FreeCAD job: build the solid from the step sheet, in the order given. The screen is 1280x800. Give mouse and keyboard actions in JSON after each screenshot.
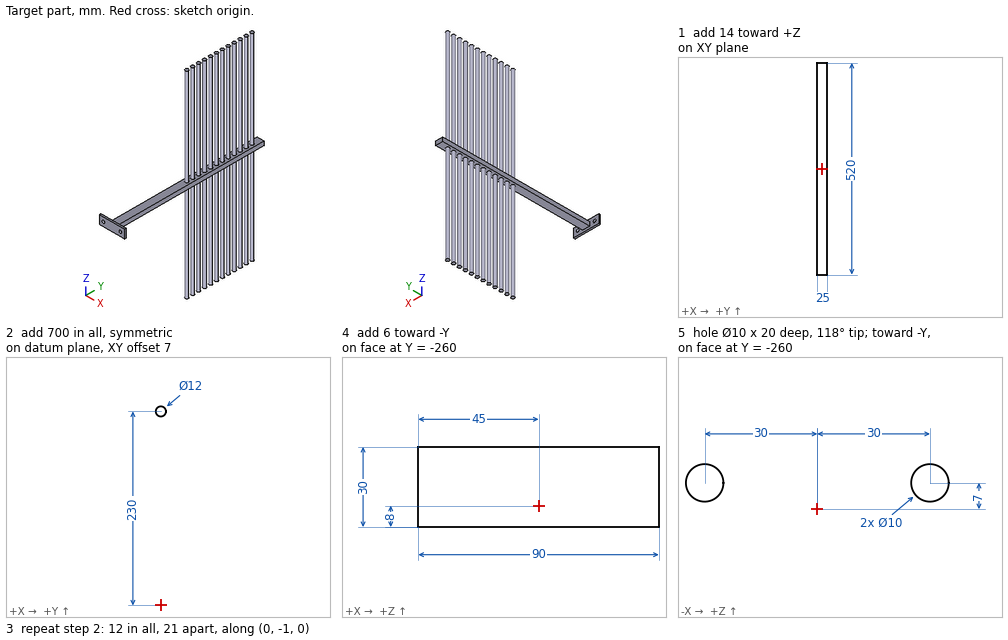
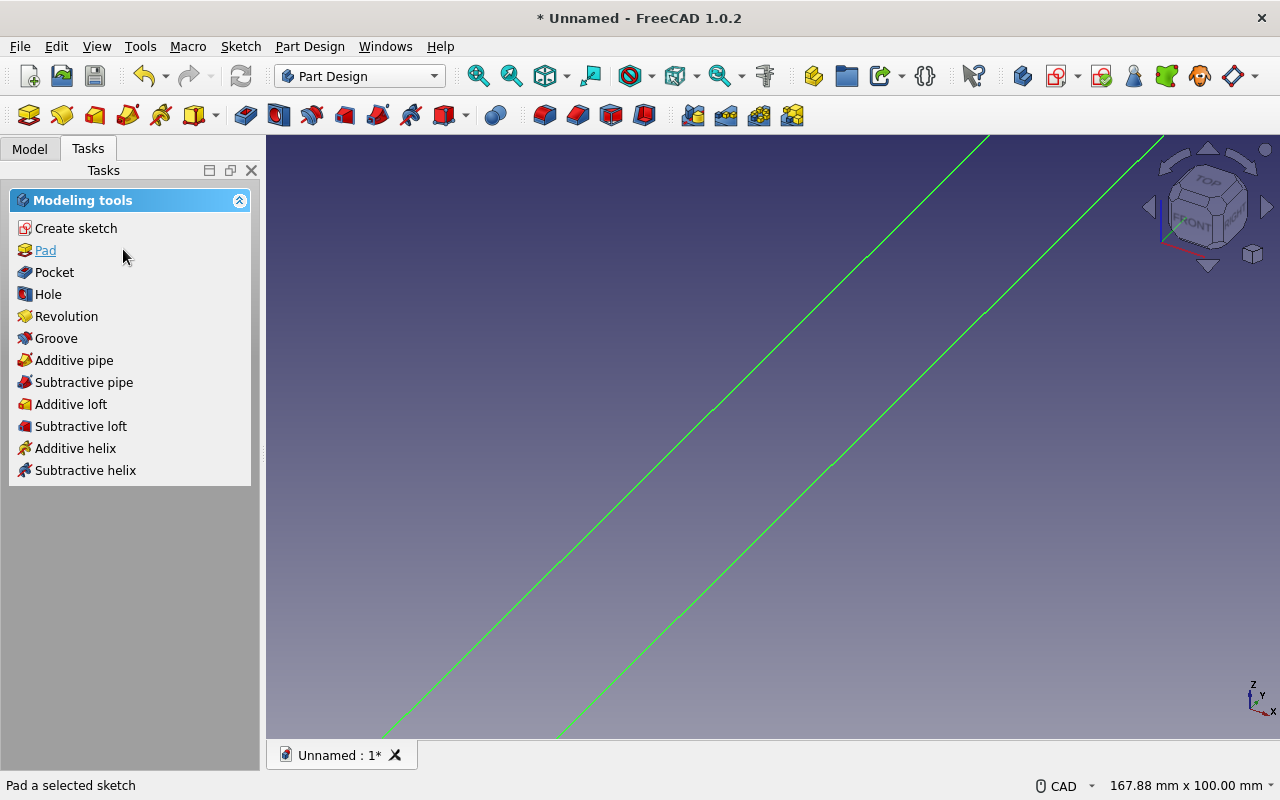
{"action": "left_click", "coordinate": [29, 116]}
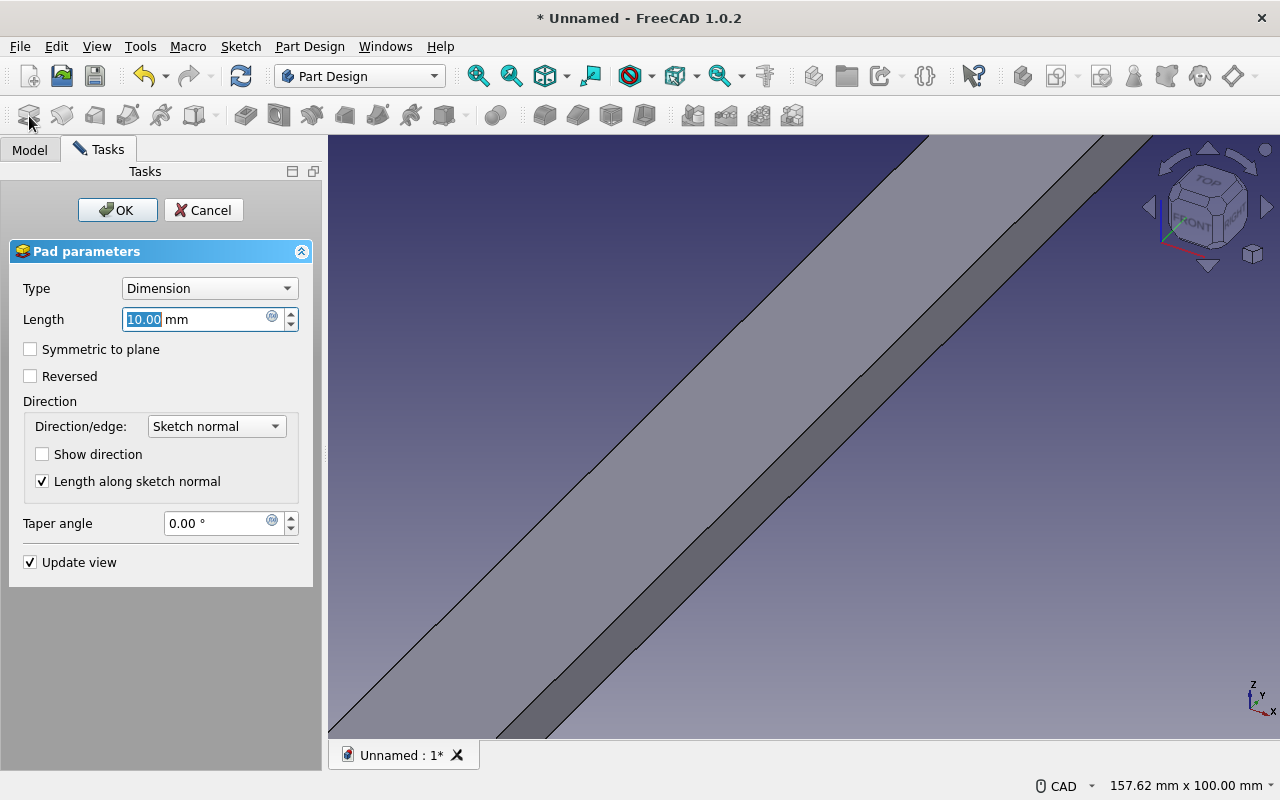
{"action": "type", "text": "14"}
{"action": "key", "text": "Tab"}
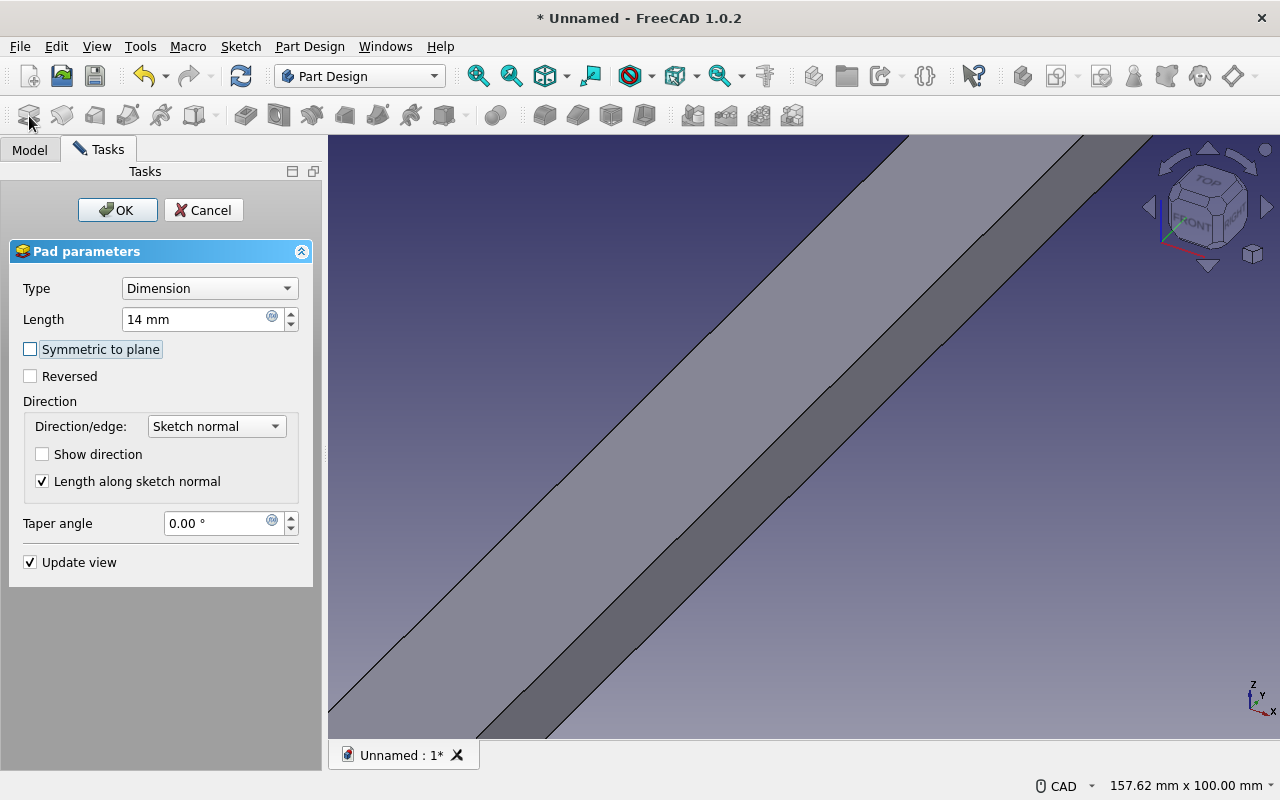
{"action": "left_click", "coordinate": [118, 210]}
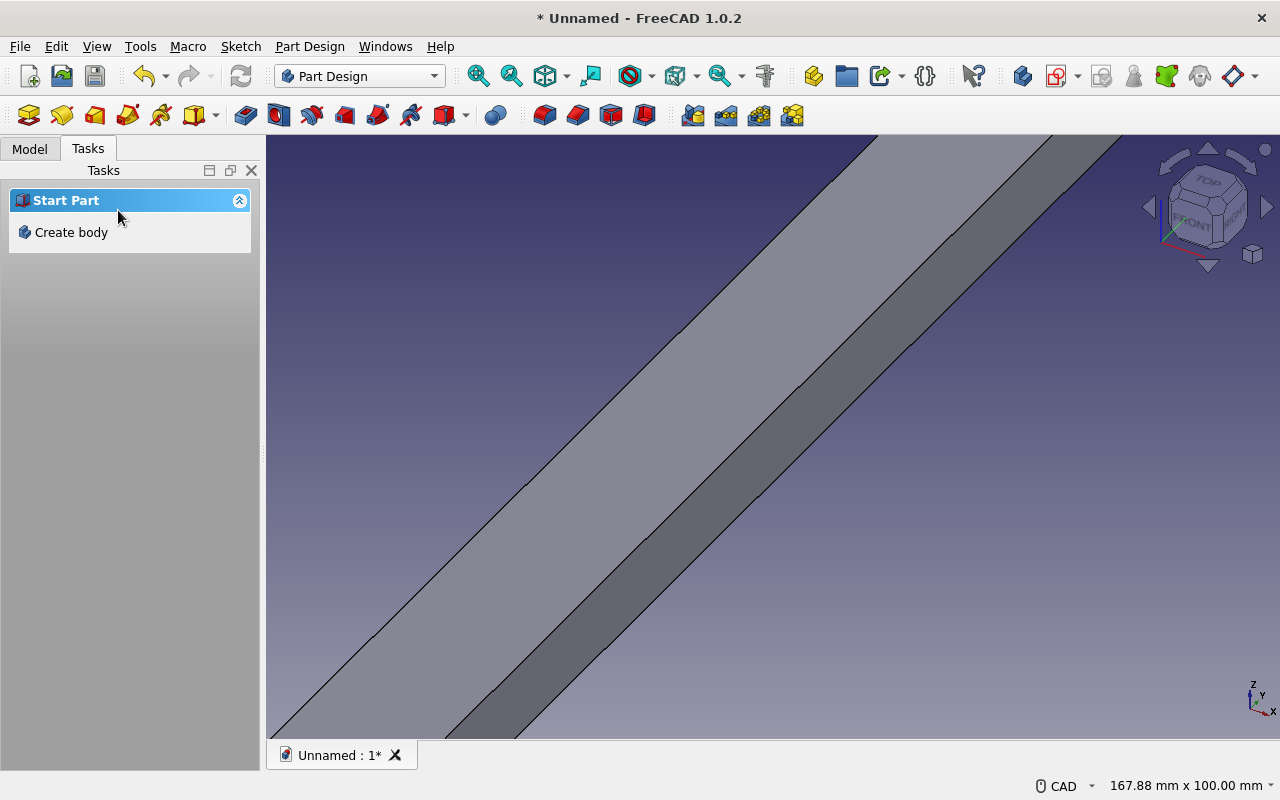
{"action": "left_click", "coordinate": [479, 76]}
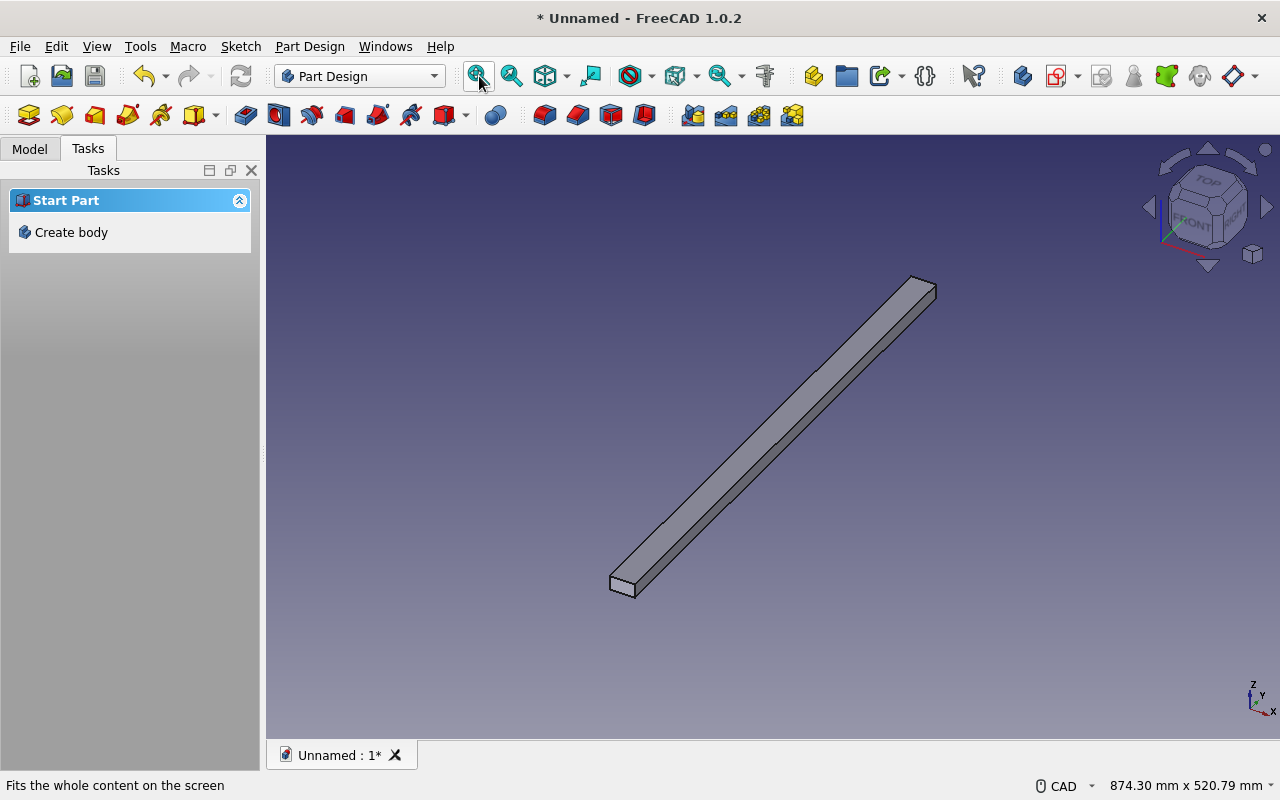
{"action": "left_click", "coordinate": [30, 148]}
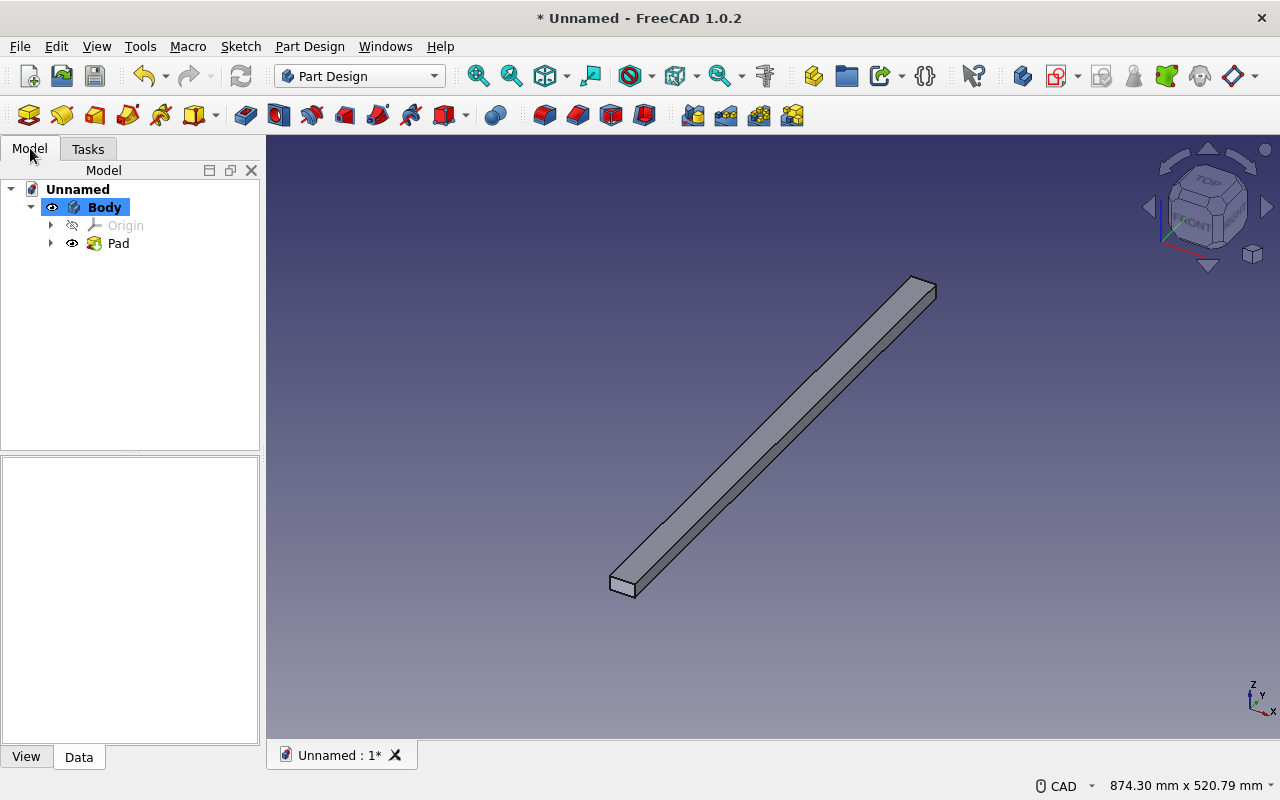
{"action": "left_click", "coordinate": [51, 225]}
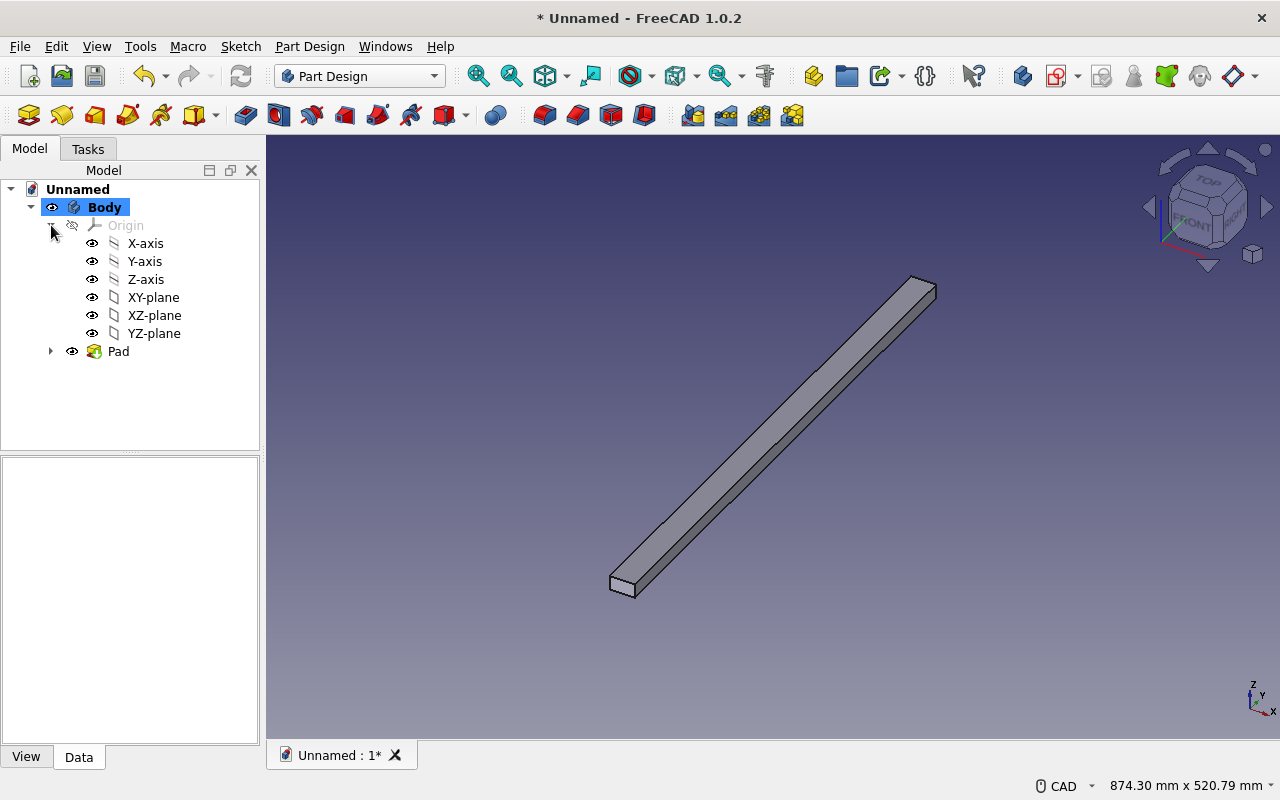
{"action": "left_click", "coordinate": [137, 297]}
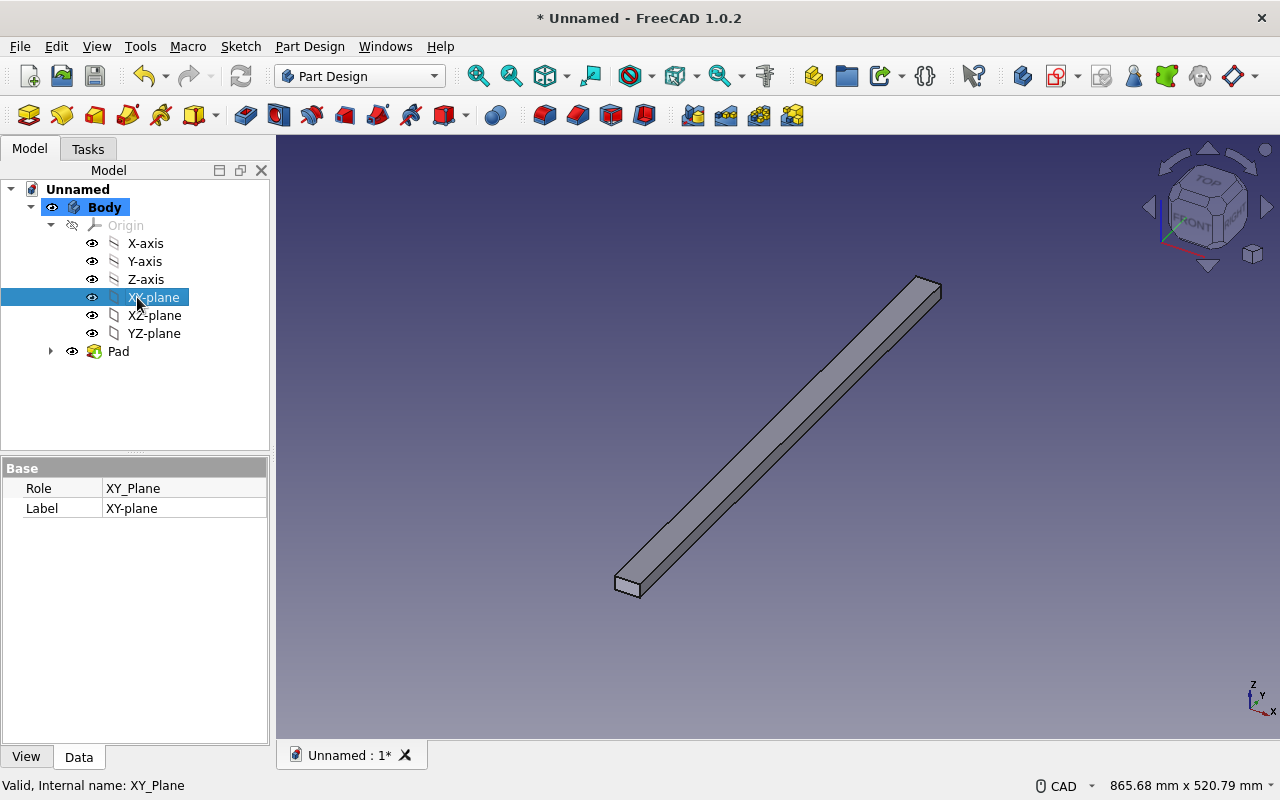
{"action": "left_click", "coordinate": [1232, 76]}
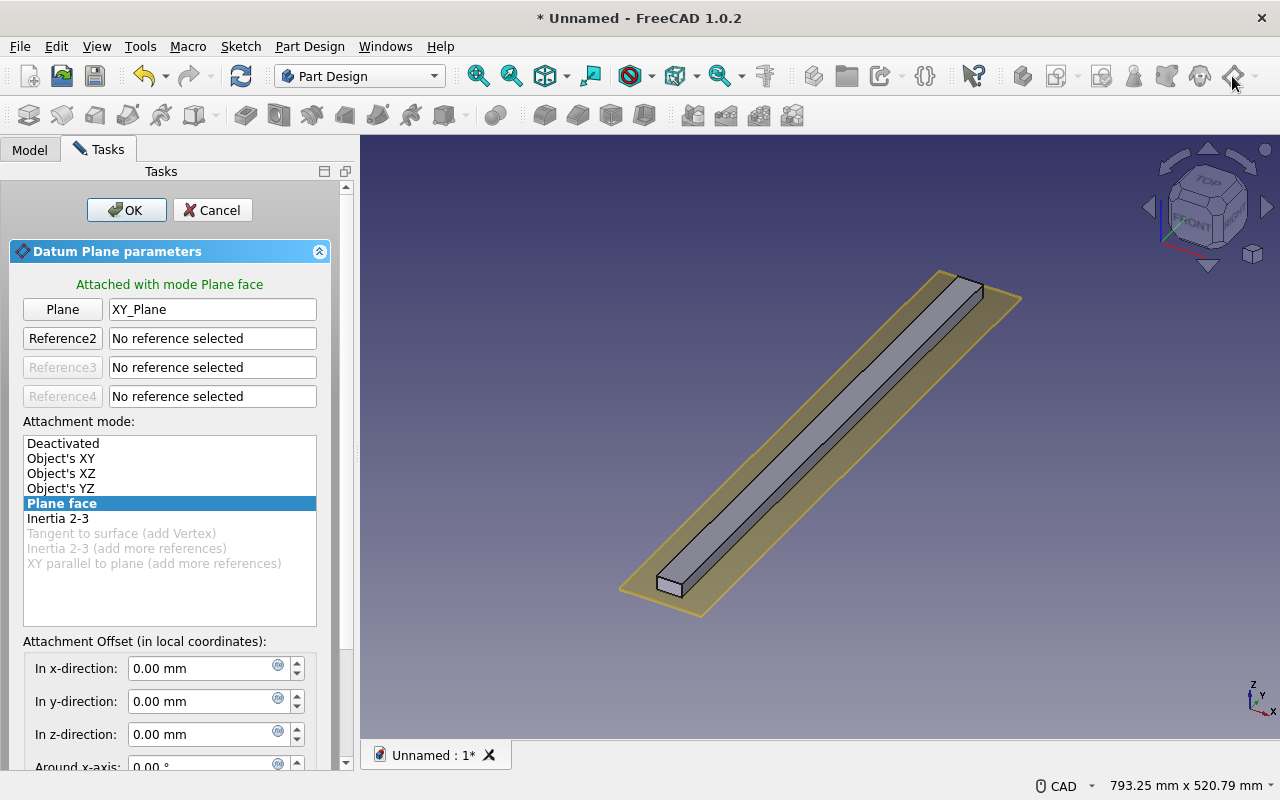
{"action": "triple_click", "coordinate": [210, 734]}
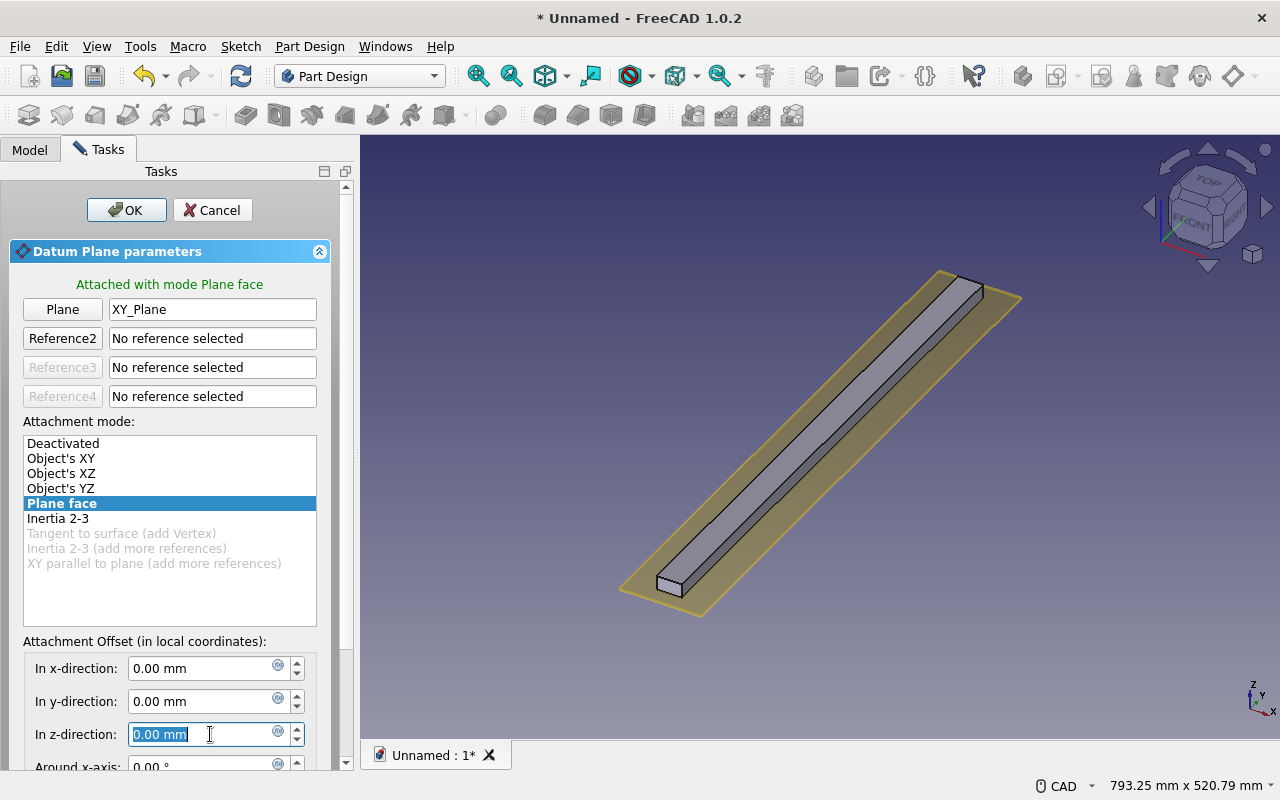
{"action": "type", "text": "7"}
{"action": "key", "text": "Tab"}